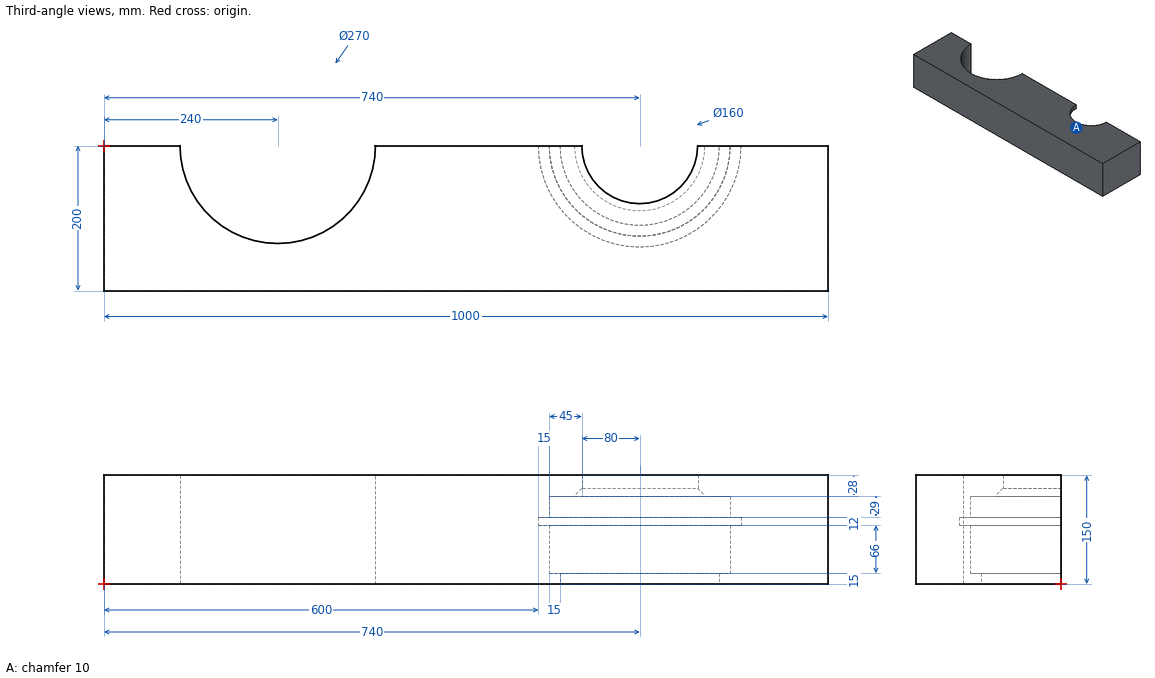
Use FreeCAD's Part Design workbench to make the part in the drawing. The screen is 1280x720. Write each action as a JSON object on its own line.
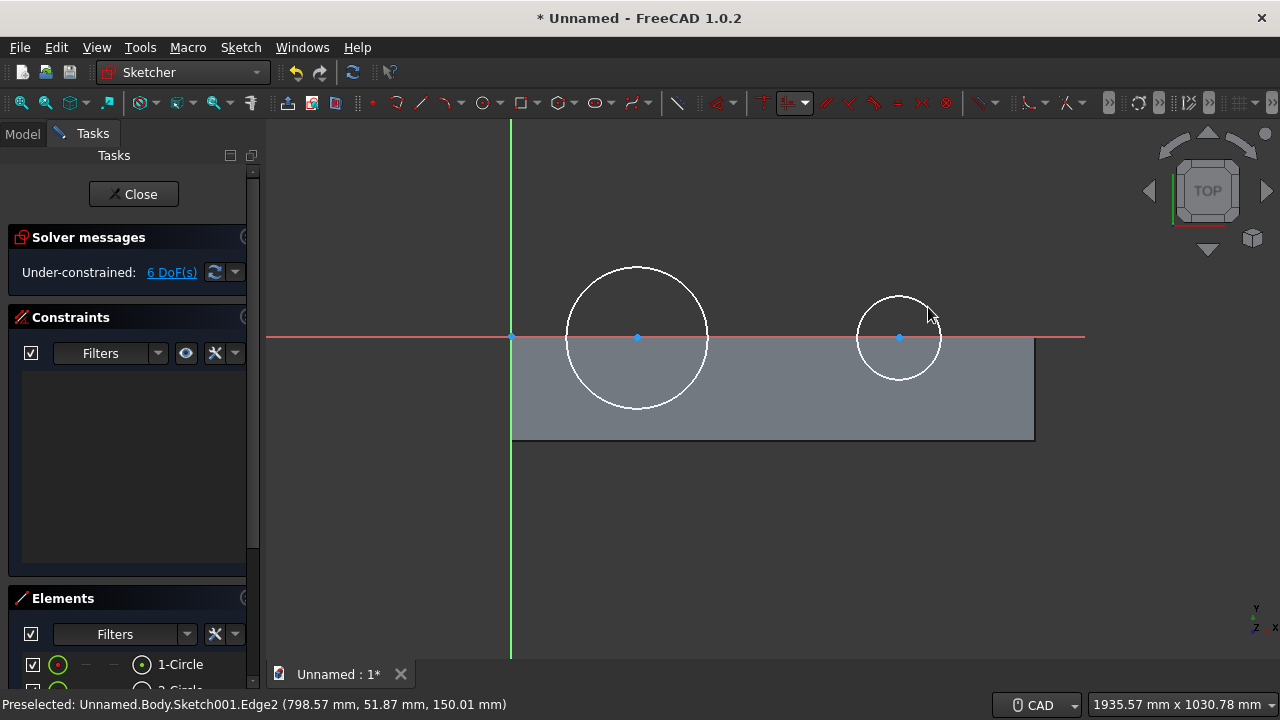
{"action": "left_click", "coordinate": [637, 338]}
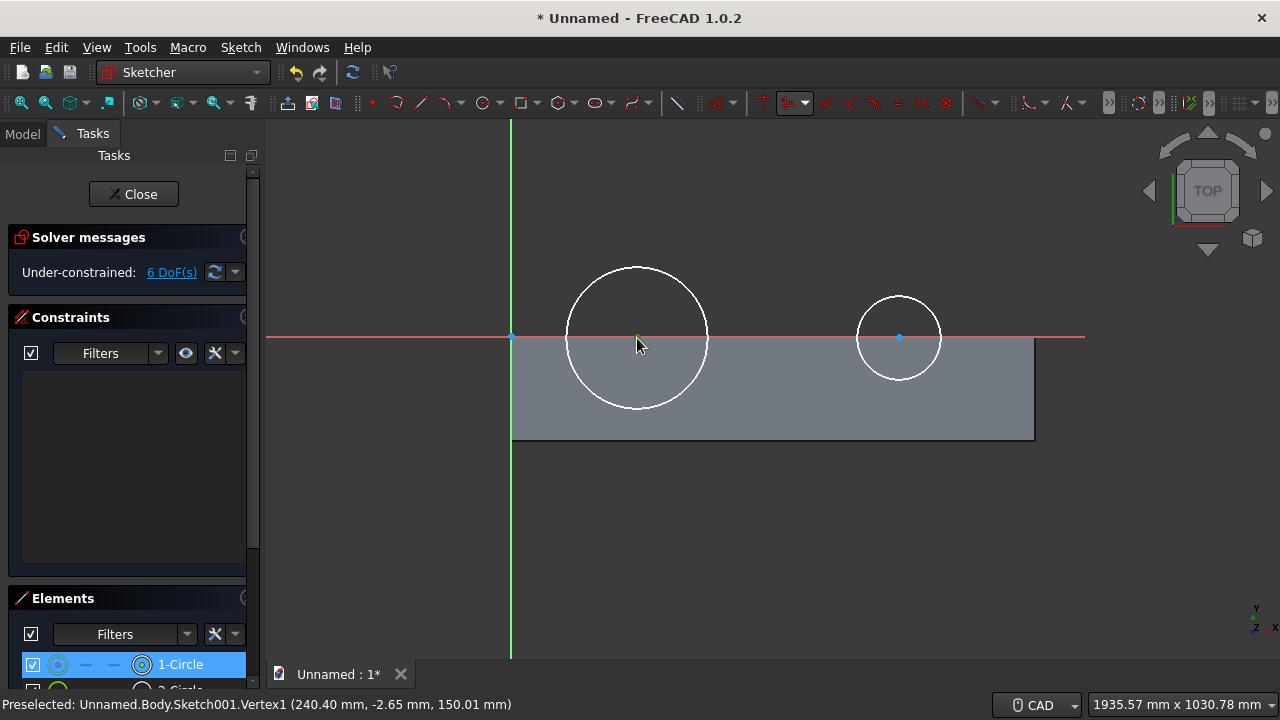
{"action": "left_click", "coordinate": [353, 337]}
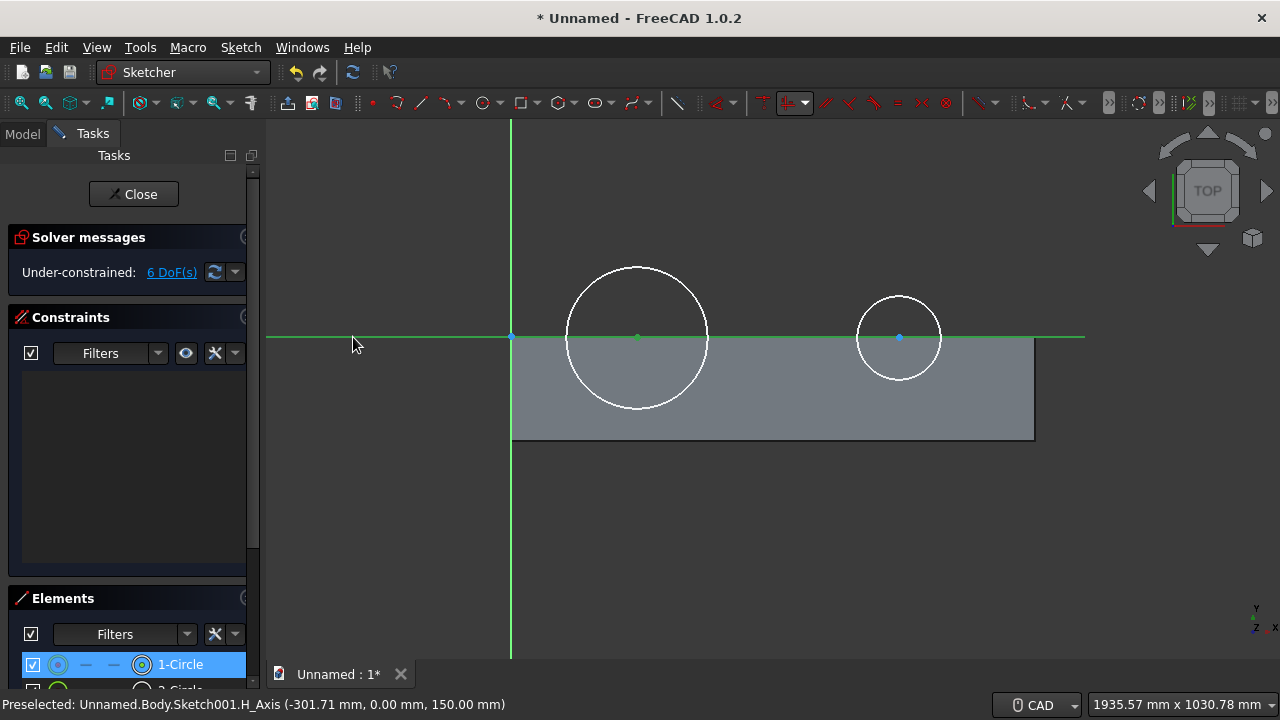
{"action": "left_click", "coordinate": [764, 104]}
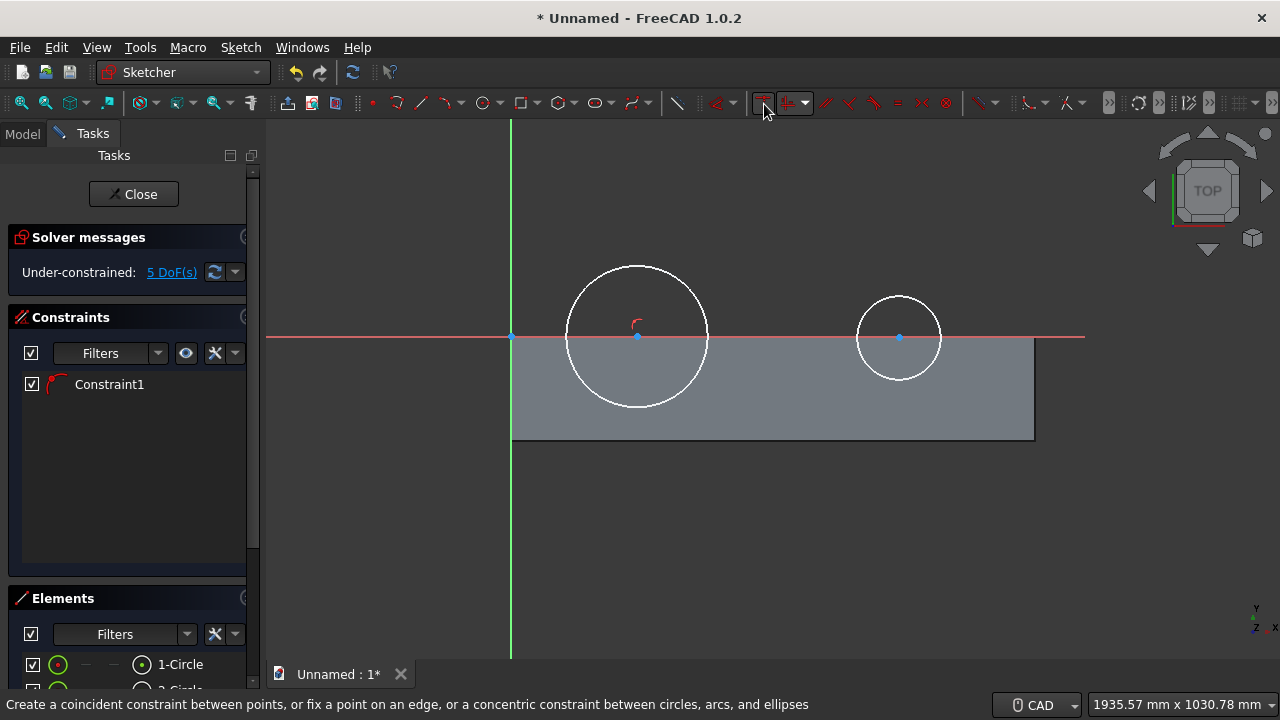
{"action": "left_click", "coordinate": [899, 338]}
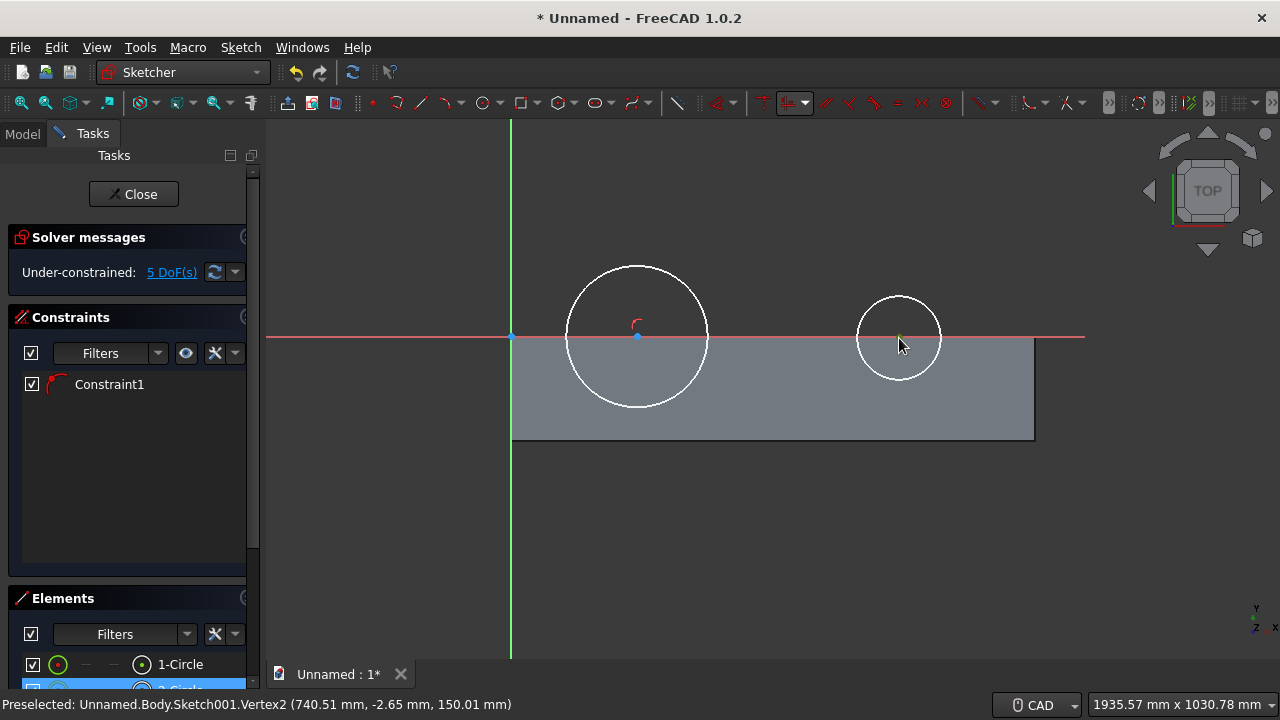
{"action": "left_click", "coordinate": [353, 337]}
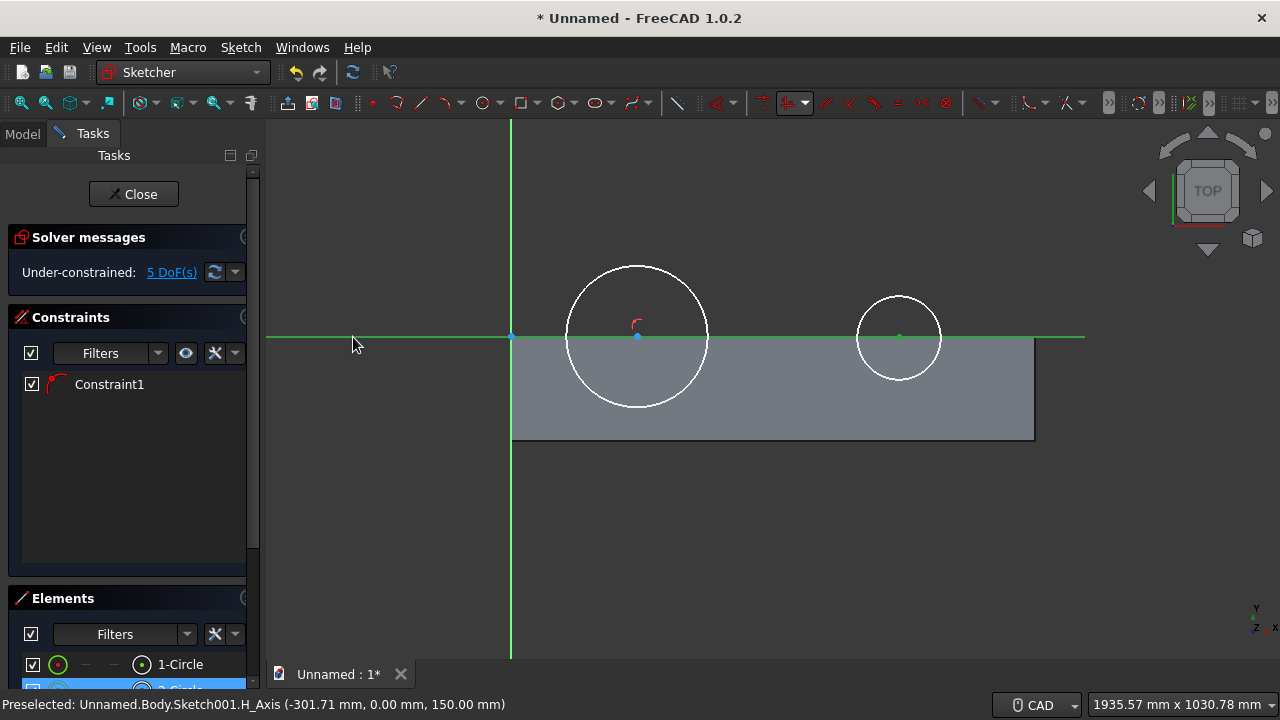
{"action": "left_click", "coordinate": [764, 104]}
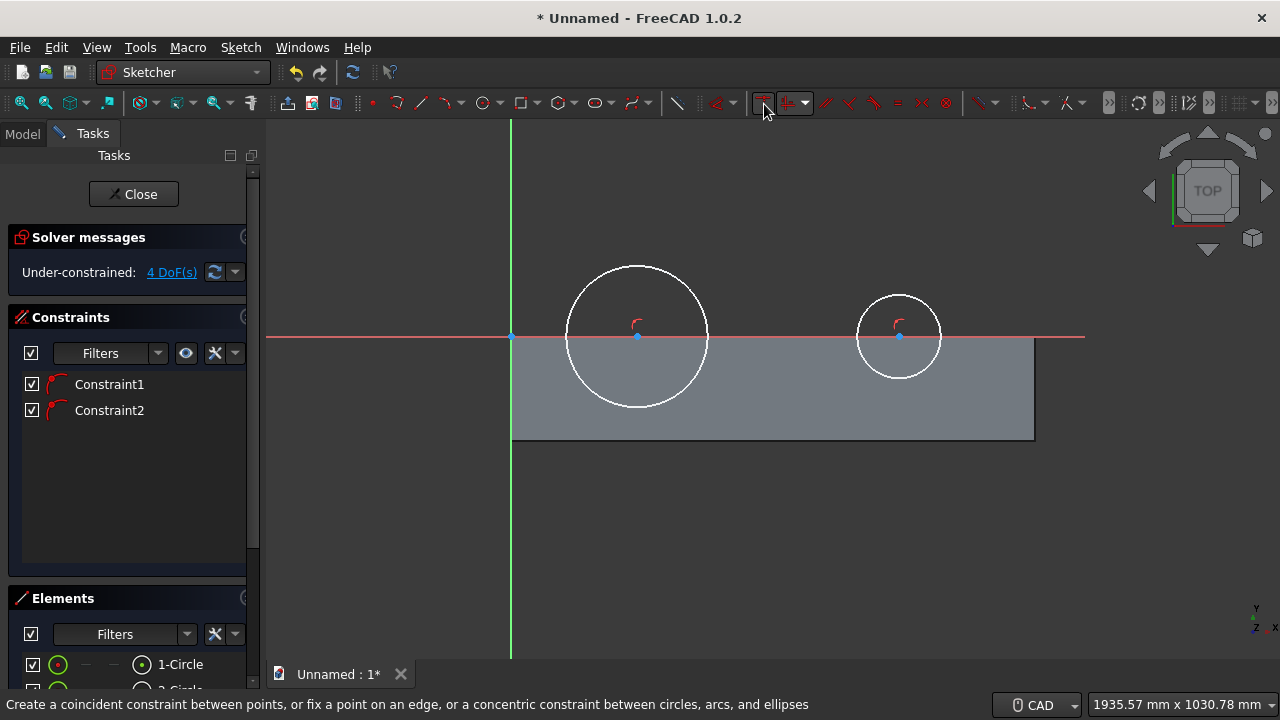
{"action": "left_click", "coordinate": [716, 104]}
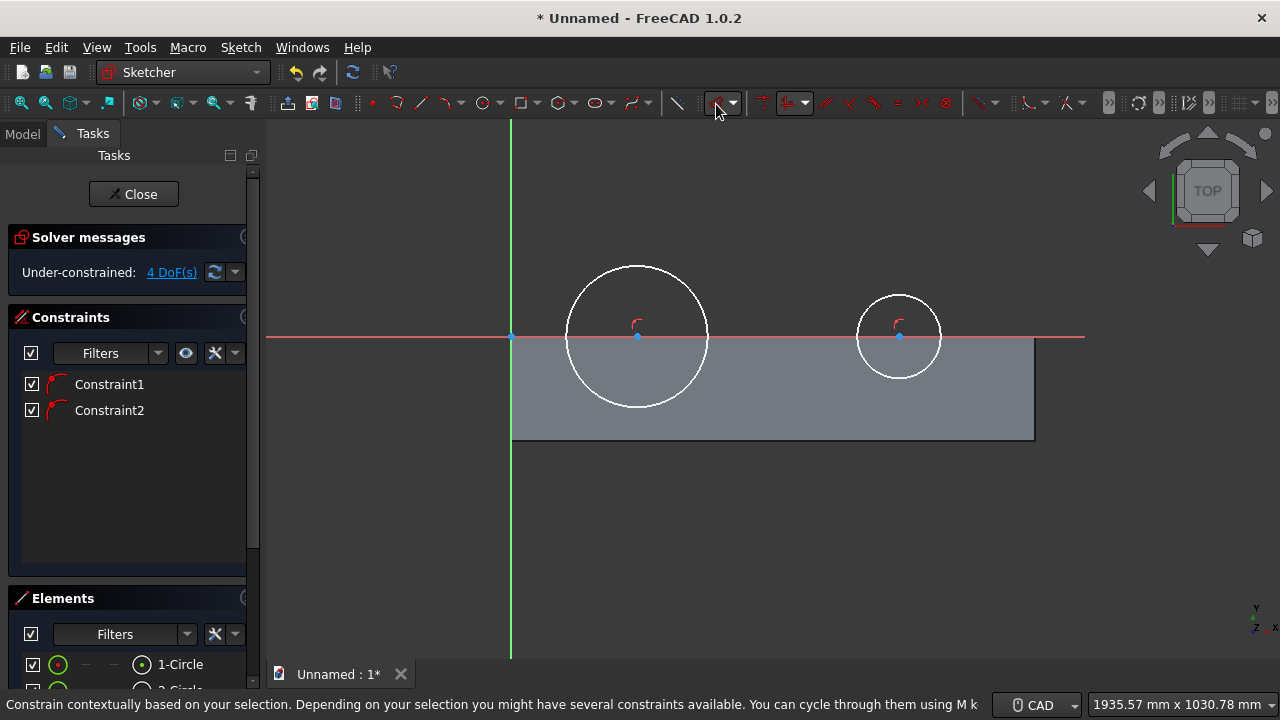
{"action": "left_click", "coordinate": [687, 286]}
{"action": "left_click", "coordinate": [709, 263]}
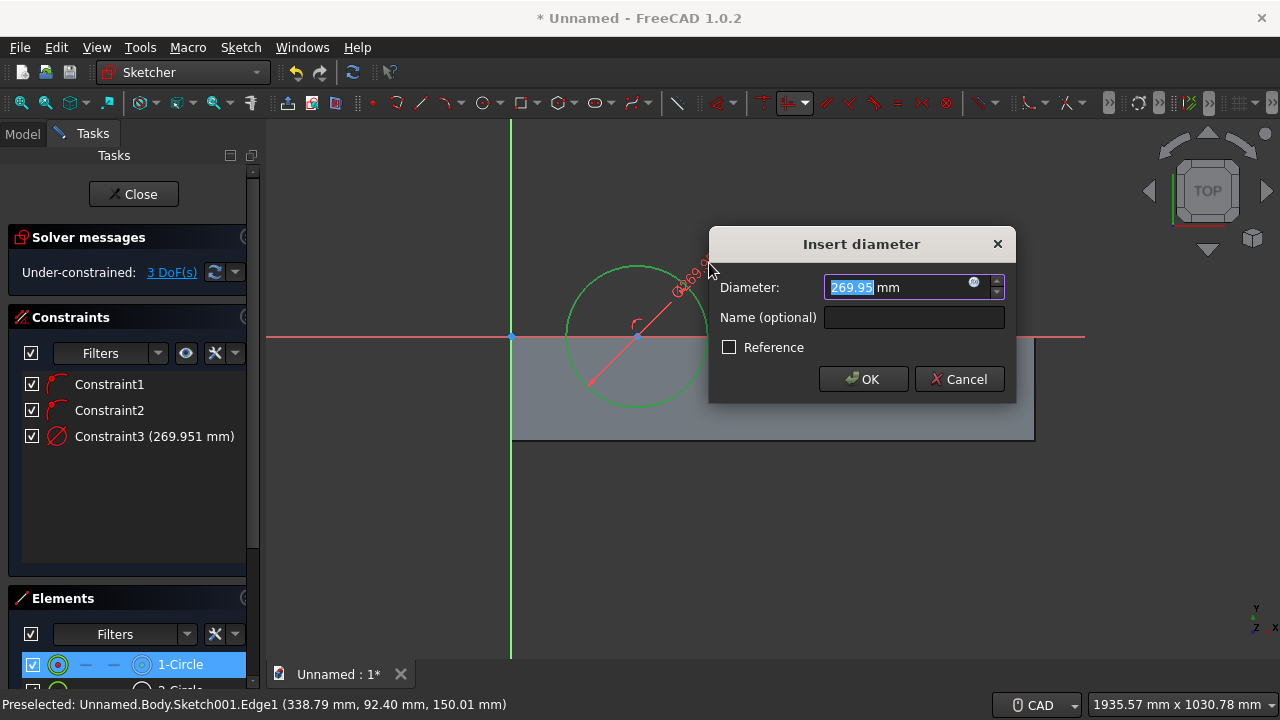
{"action": "type", "text": "270"}
{"action": "key", "text": "Return"}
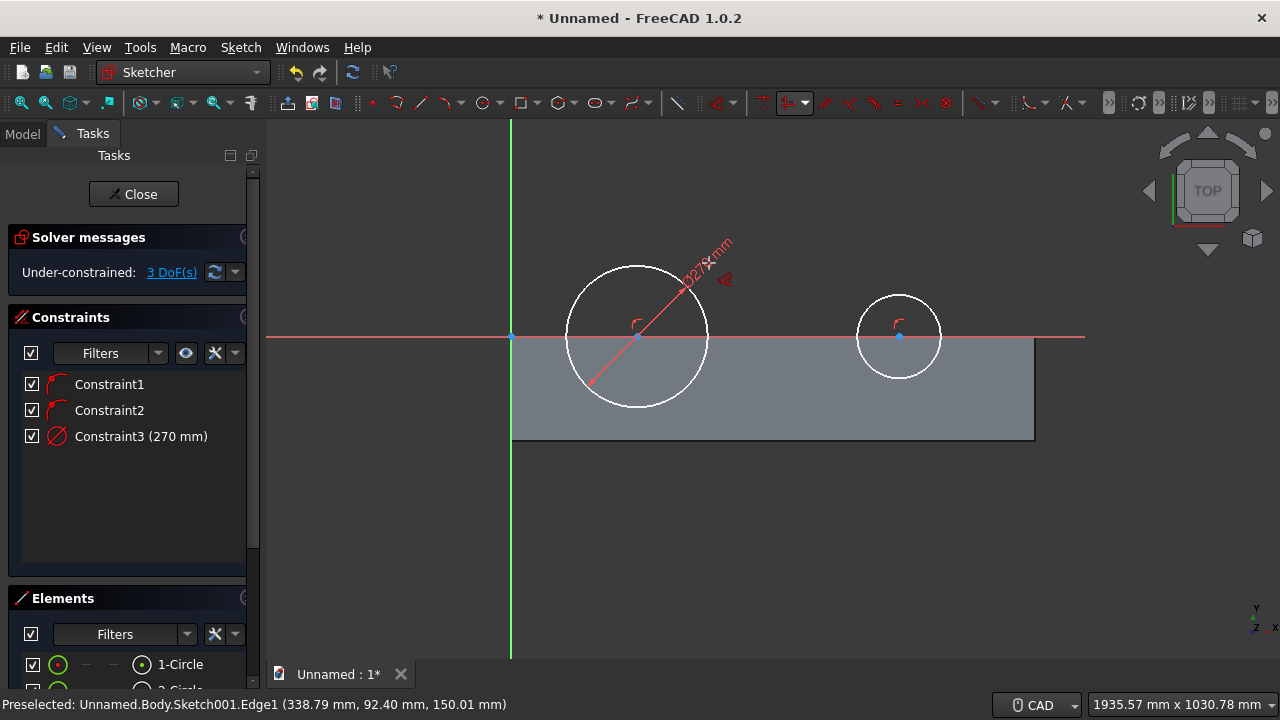
{"action": "left_click", "coordinate": [928, 307]}
{"action": "left_click", "coordinate": [950, 284]}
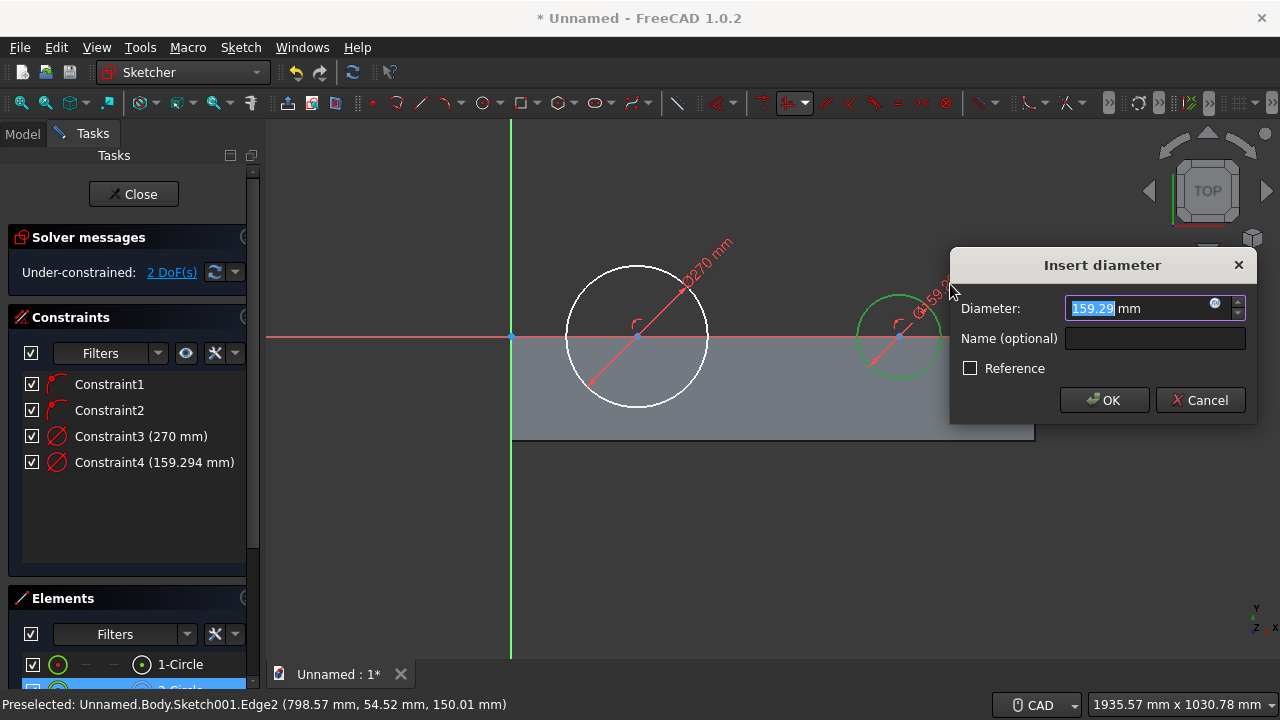
{"action": "type", "text": "160"}
{"action": "key", "text": "Return"}